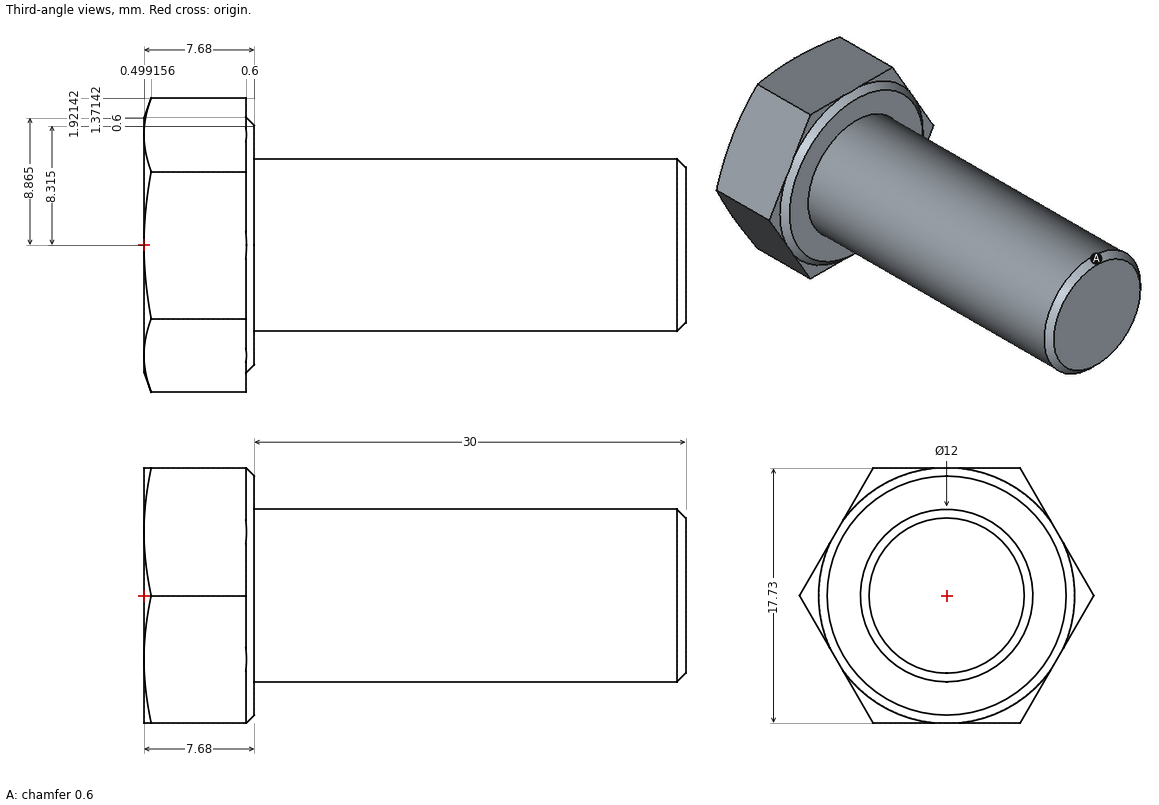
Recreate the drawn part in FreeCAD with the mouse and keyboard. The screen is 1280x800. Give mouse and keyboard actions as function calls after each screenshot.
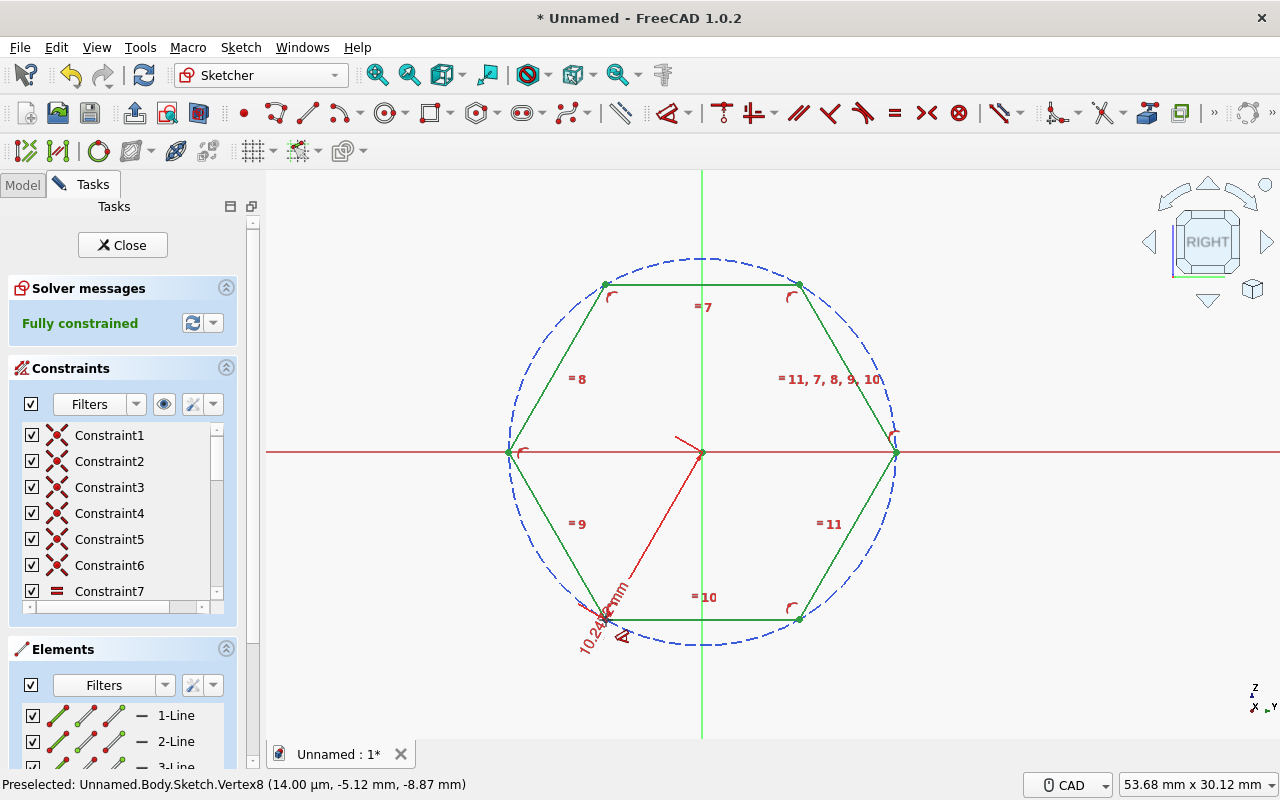
click(799, 285)
click(572, 375)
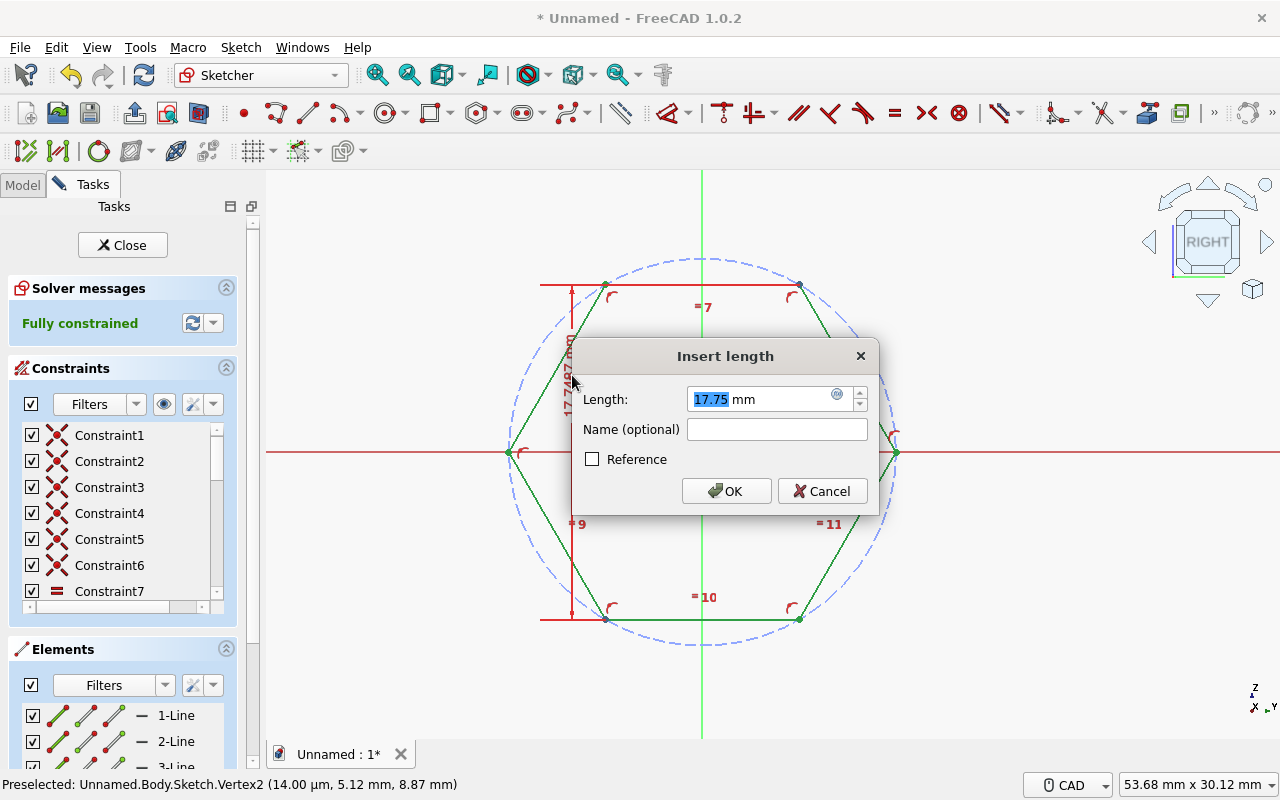
text(17.73)
key(Return)
key(Escape)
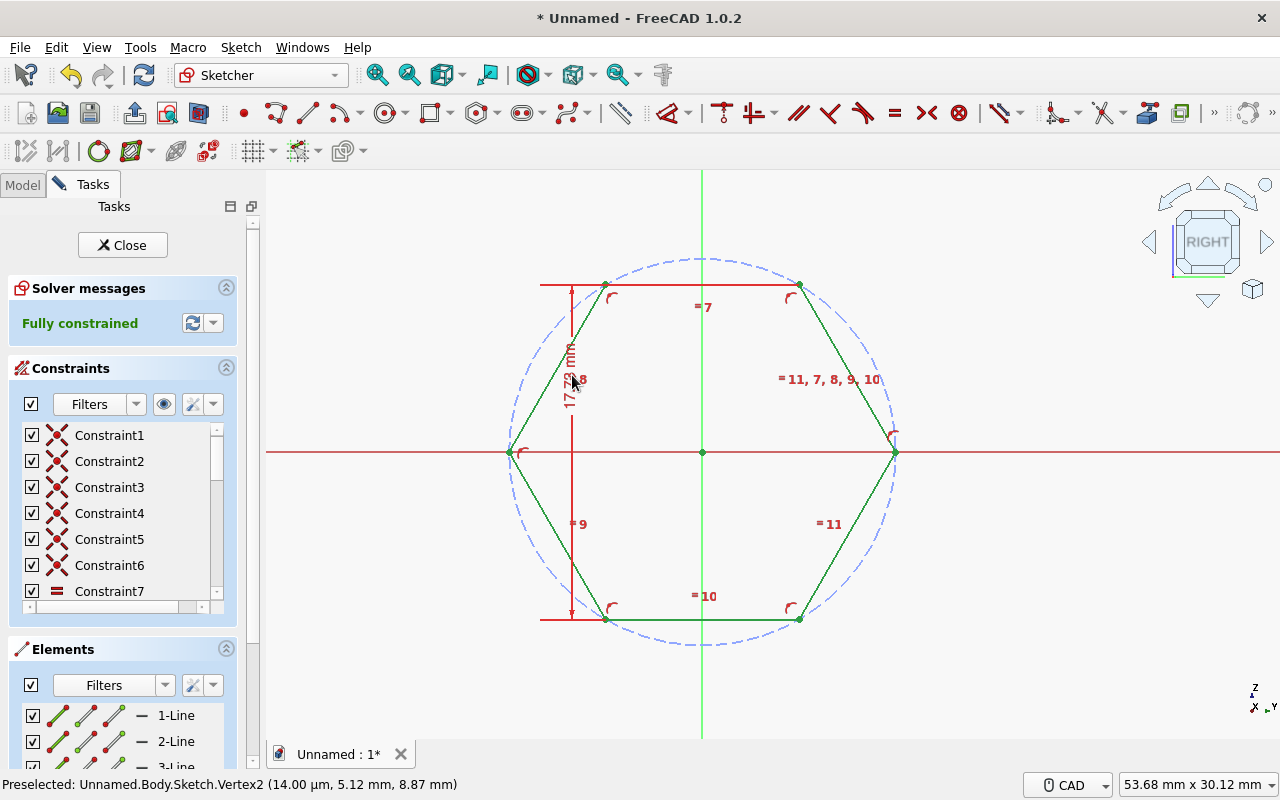
click(123, 245)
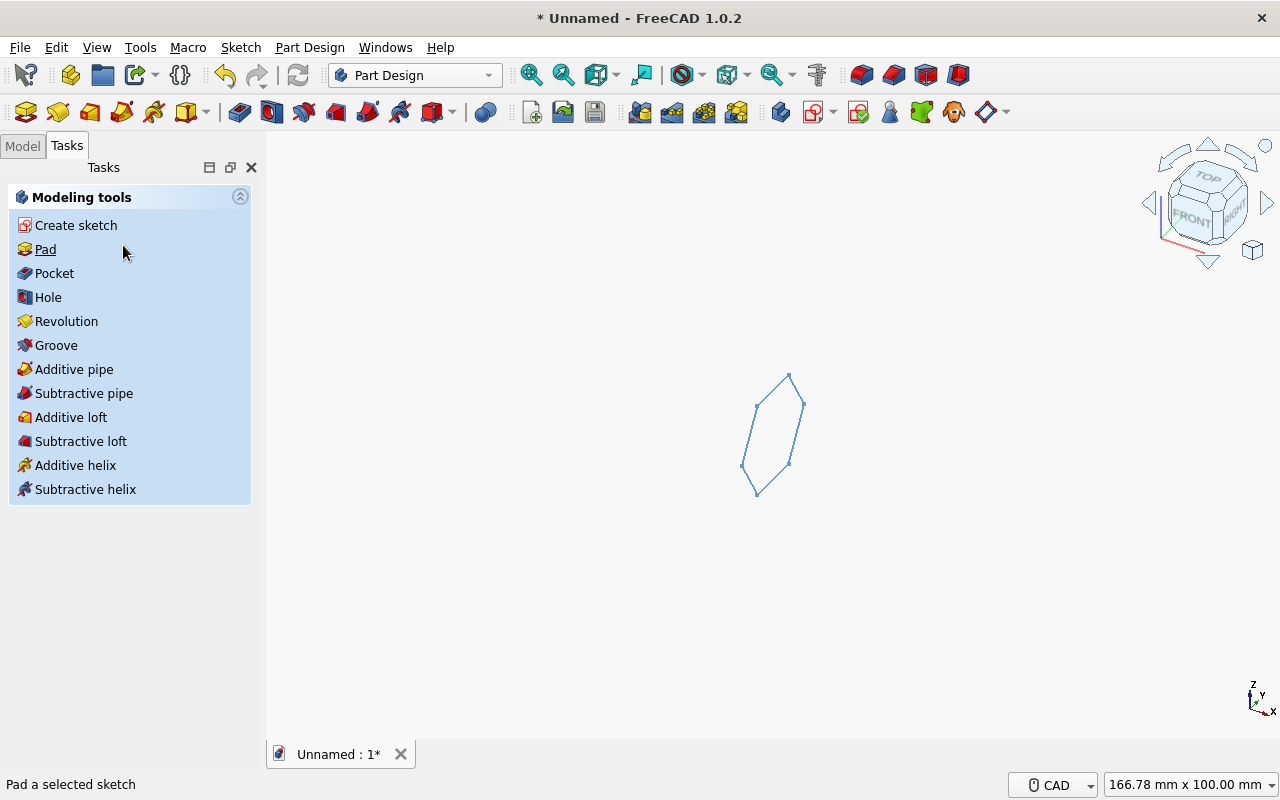
click(26, 112)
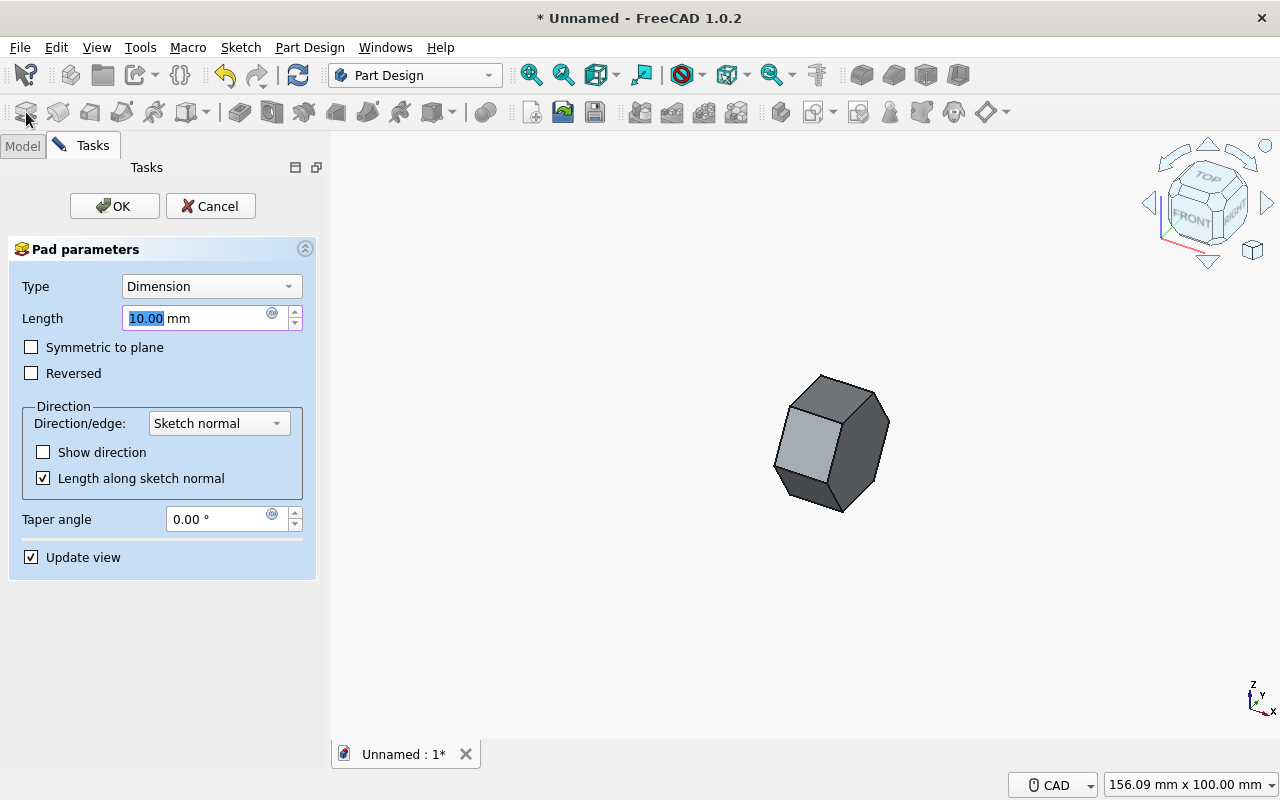
text(7.68)
key(Tab)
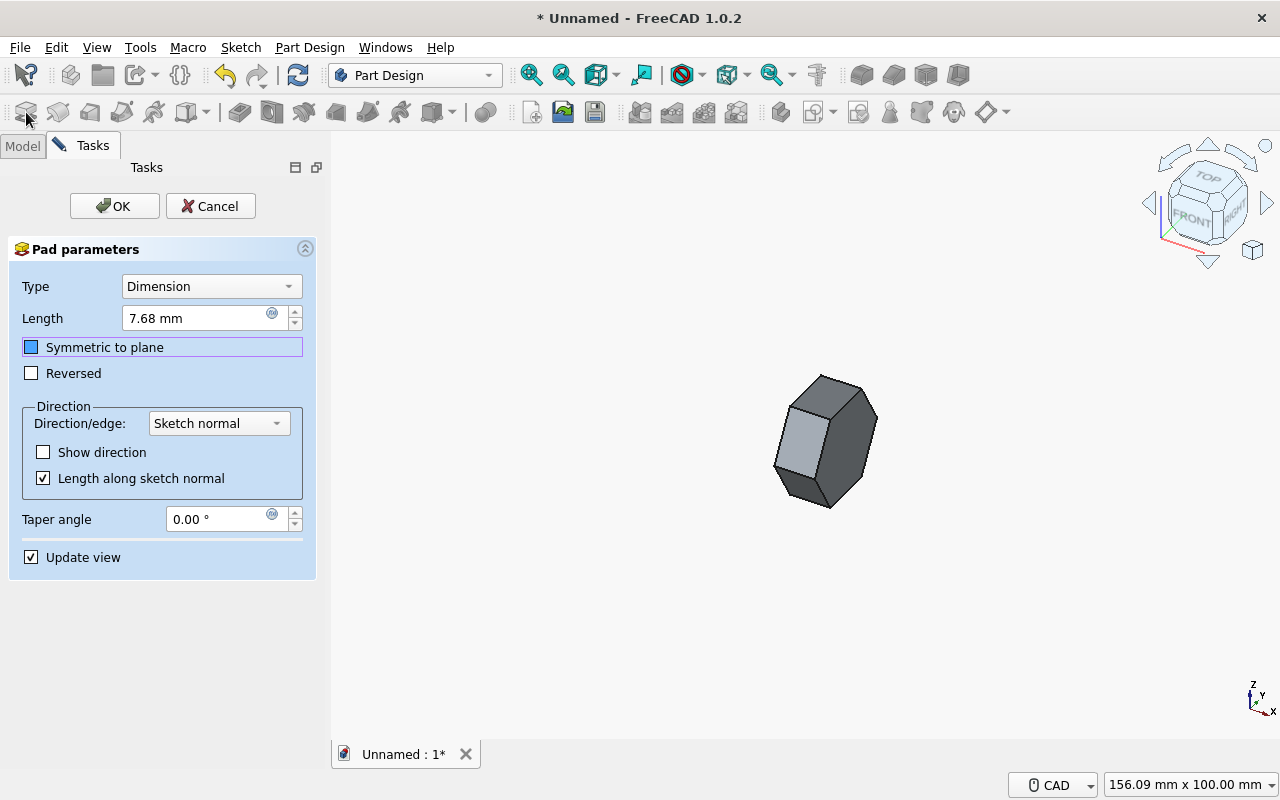
click(115, 206)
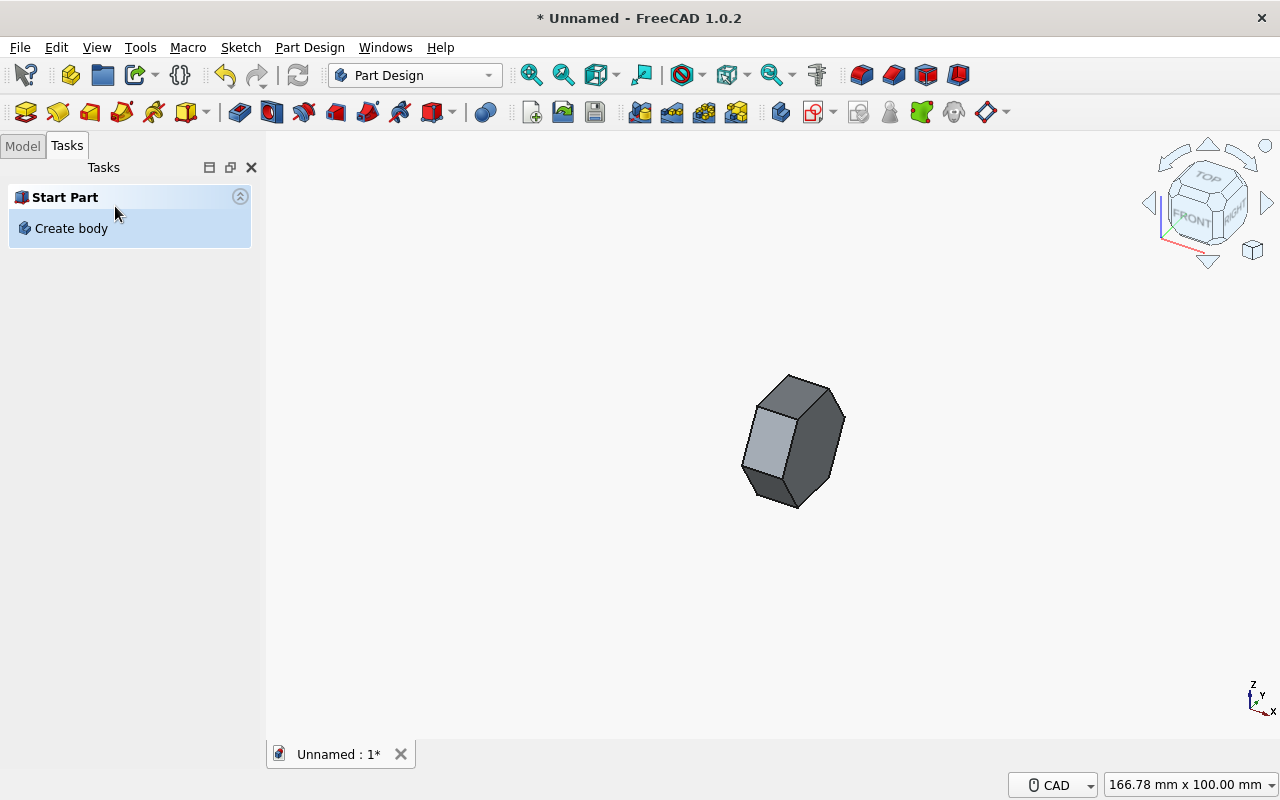
key(v)
key(f)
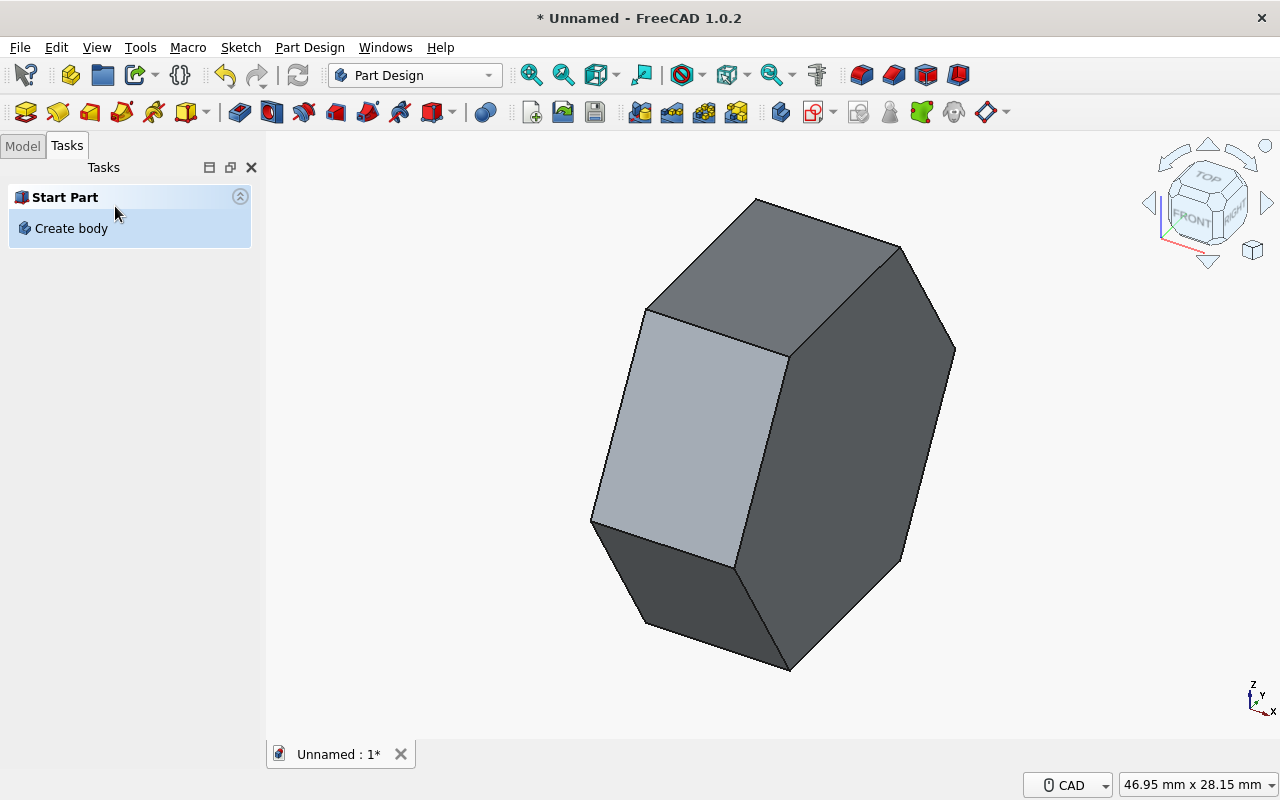
click(814, 112)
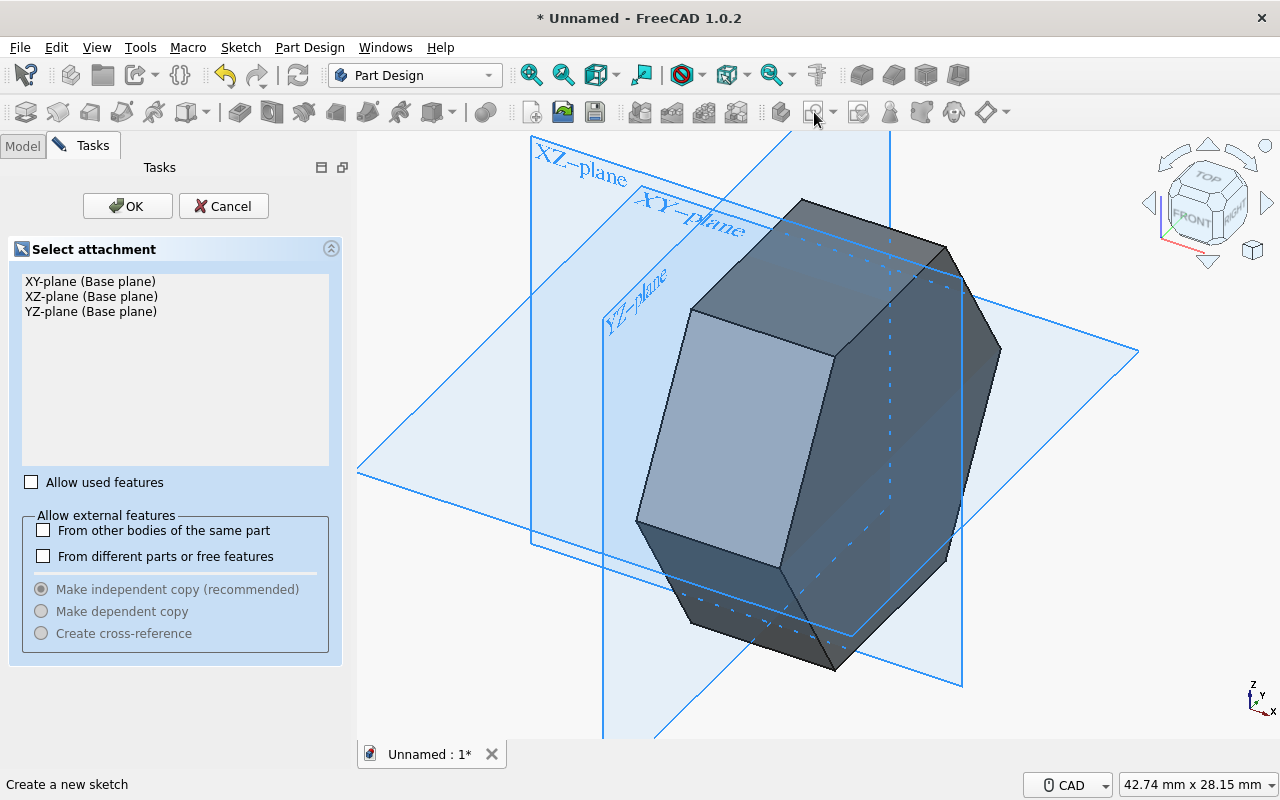
click(82, 282)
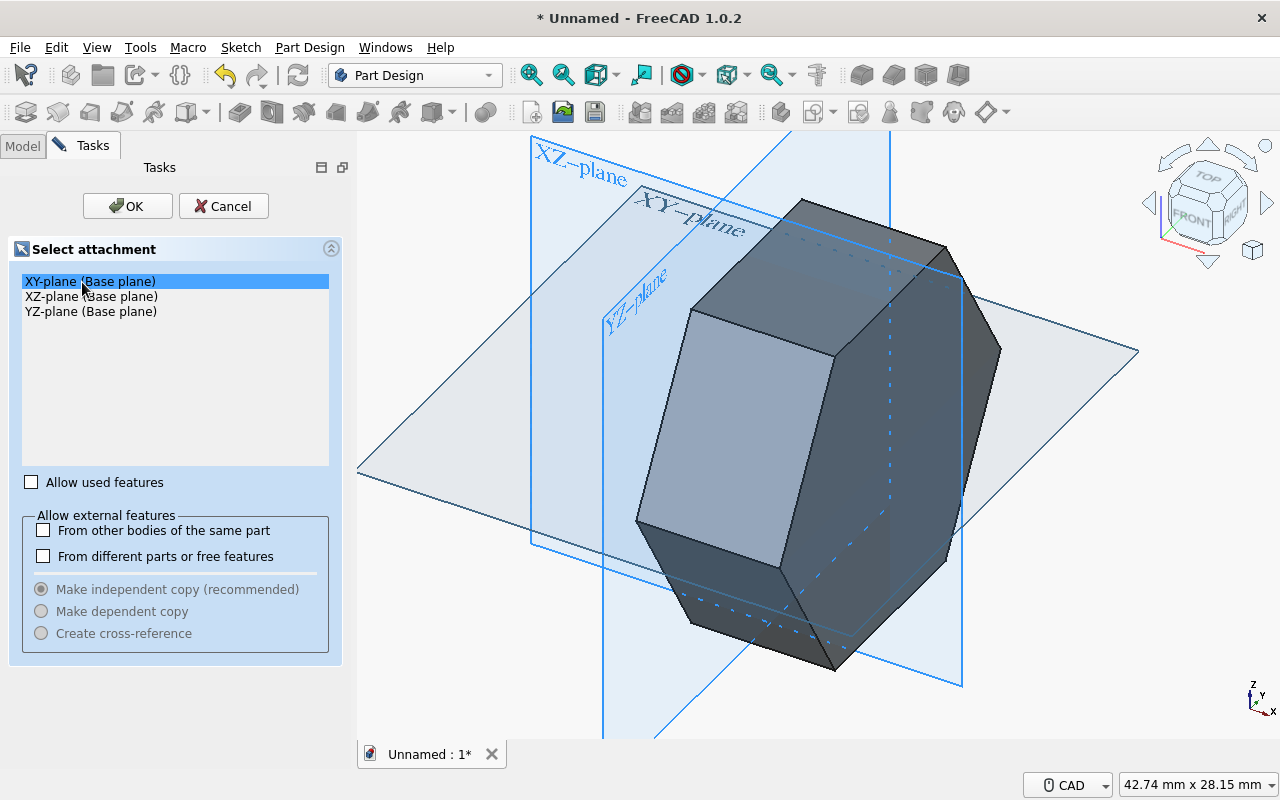
click(128, 206)